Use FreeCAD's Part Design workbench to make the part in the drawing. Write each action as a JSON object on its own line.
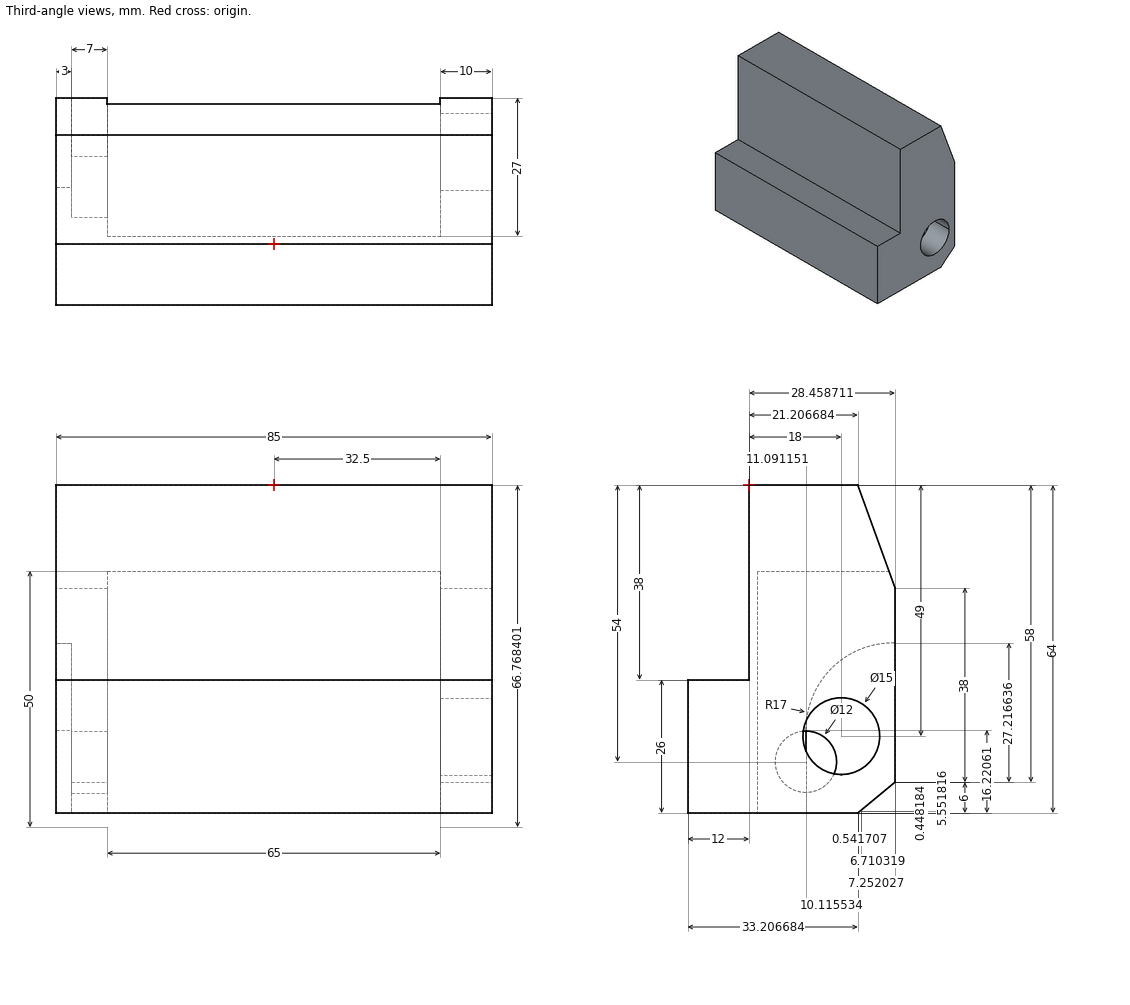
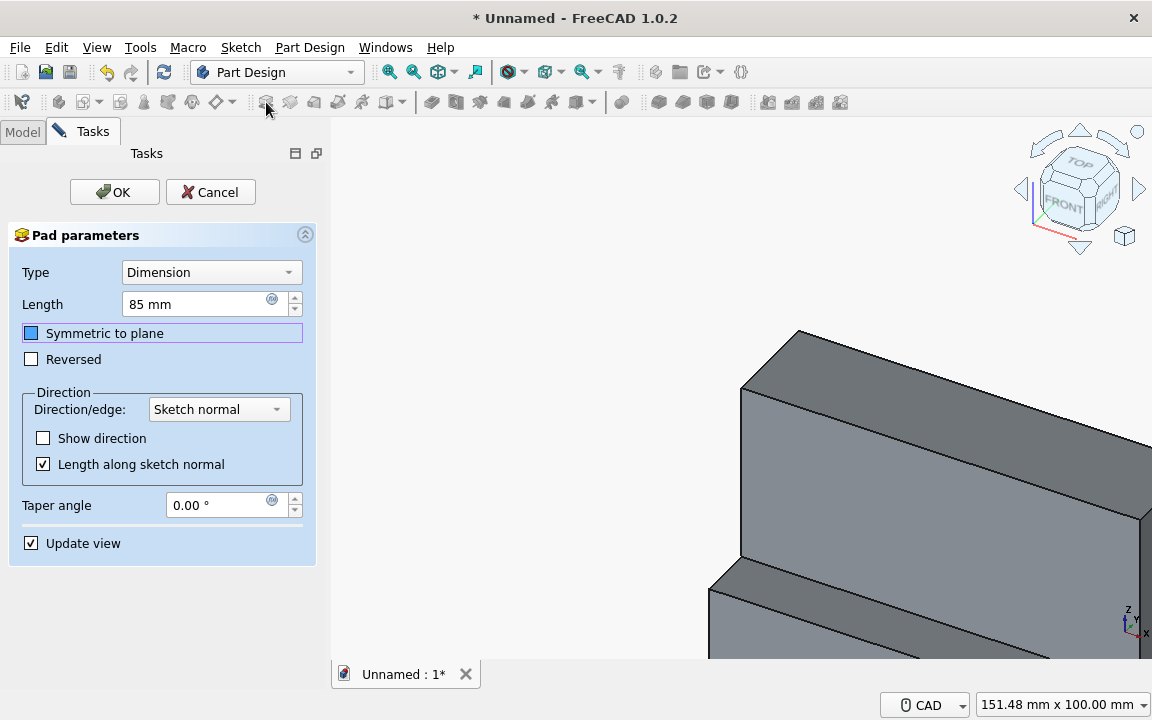
{"action": "left_click", "coordinate": [30, 333]}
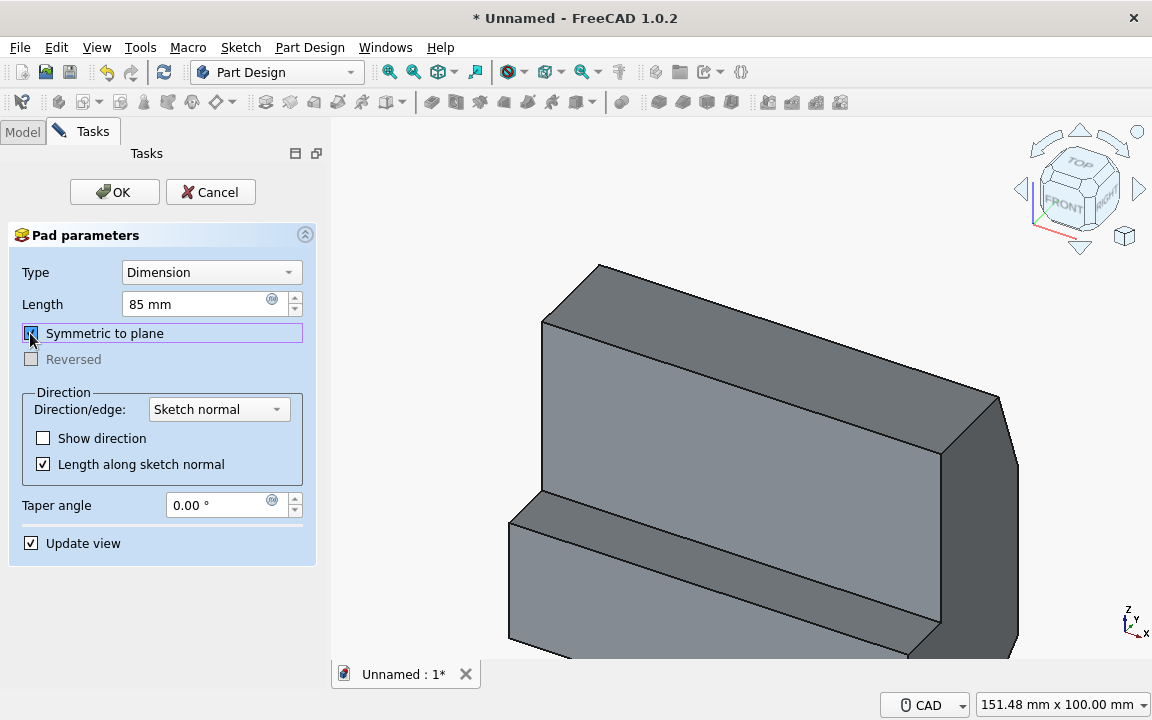
{"action": "left_click", "coordinate": [115, 192]}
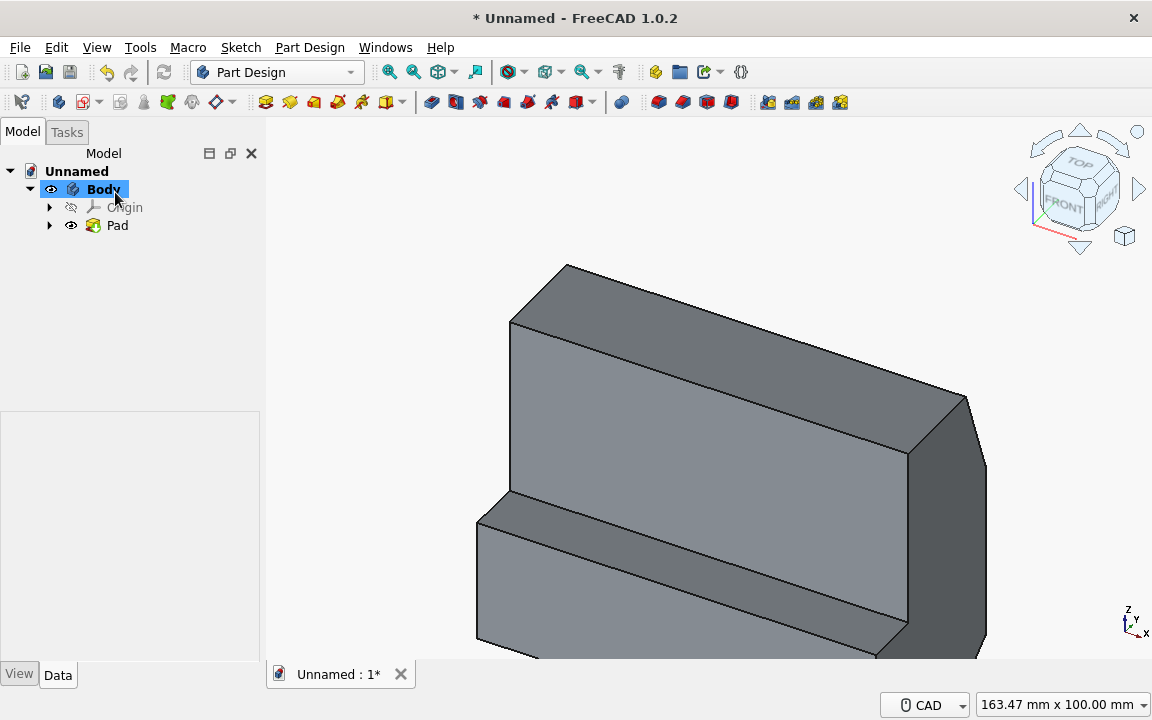
{"action": "left_click", "coordinate": [390, 72]}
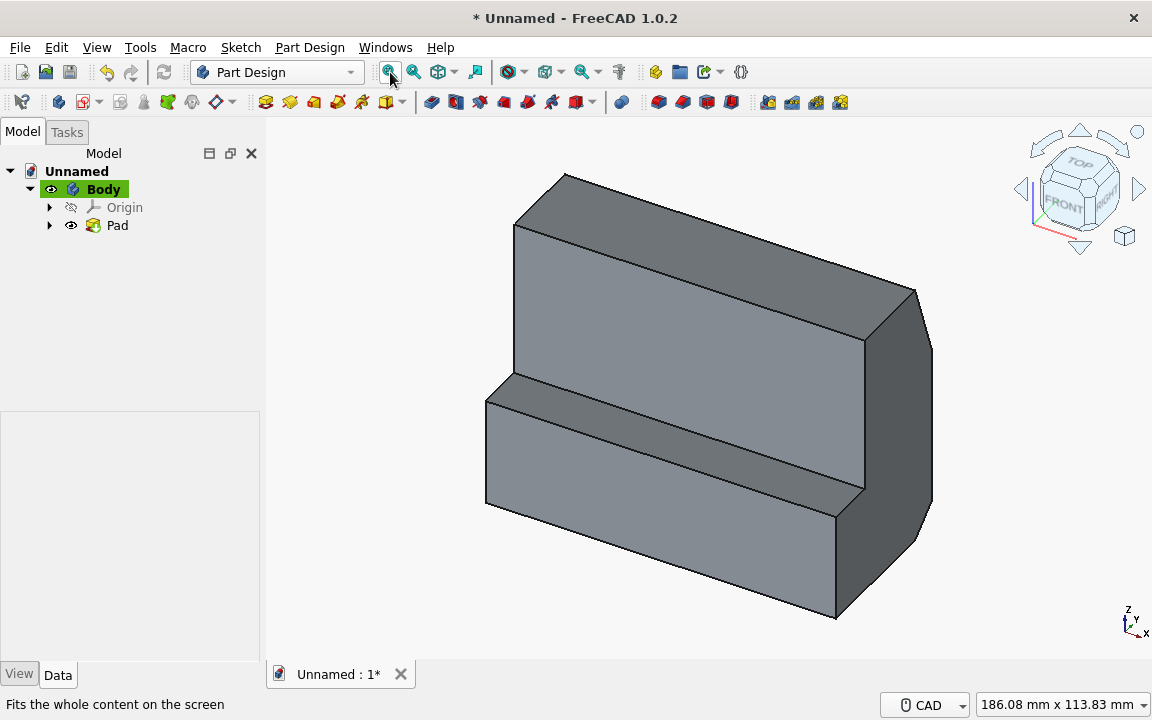
{"action": "key", "text": "4"}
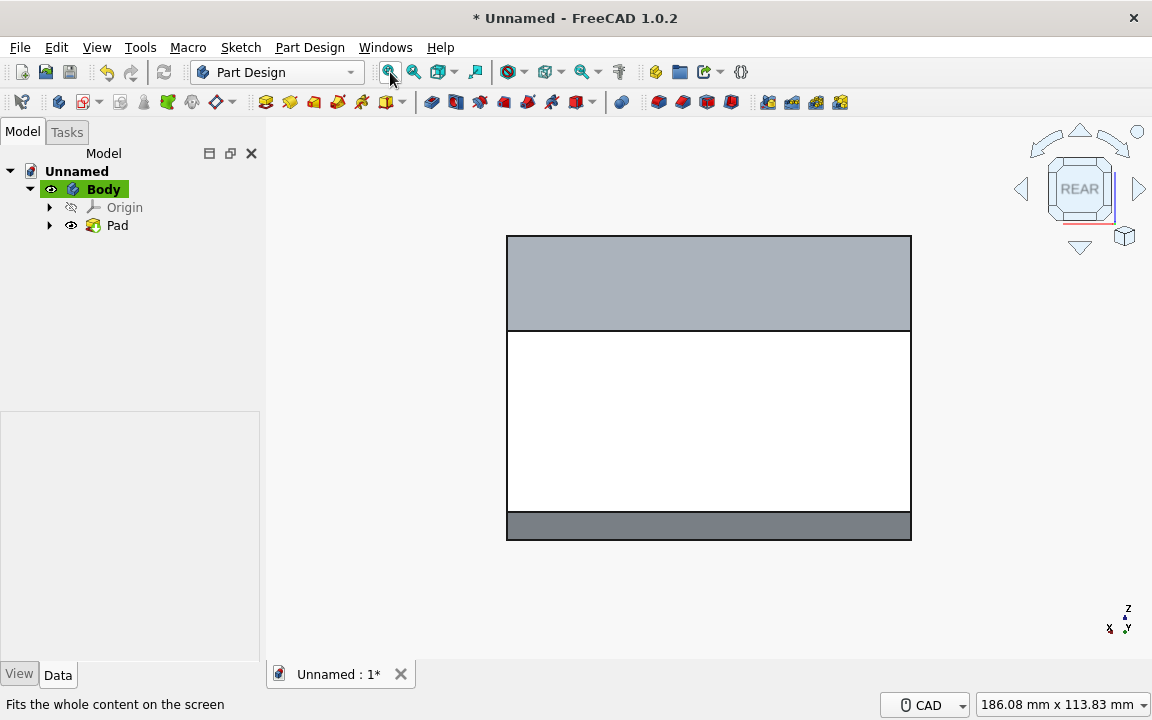
{"action": "left_click", "coordinate": [651, 420]}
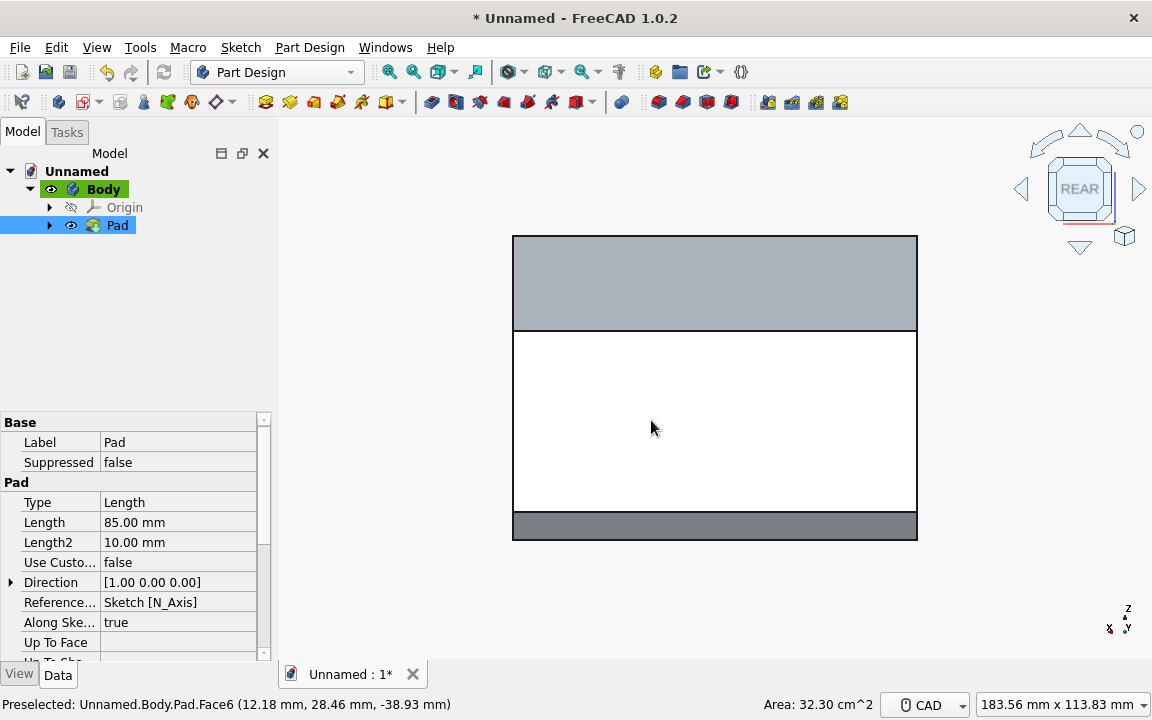
{"action": "left_click", "coordinate": [84, 102]}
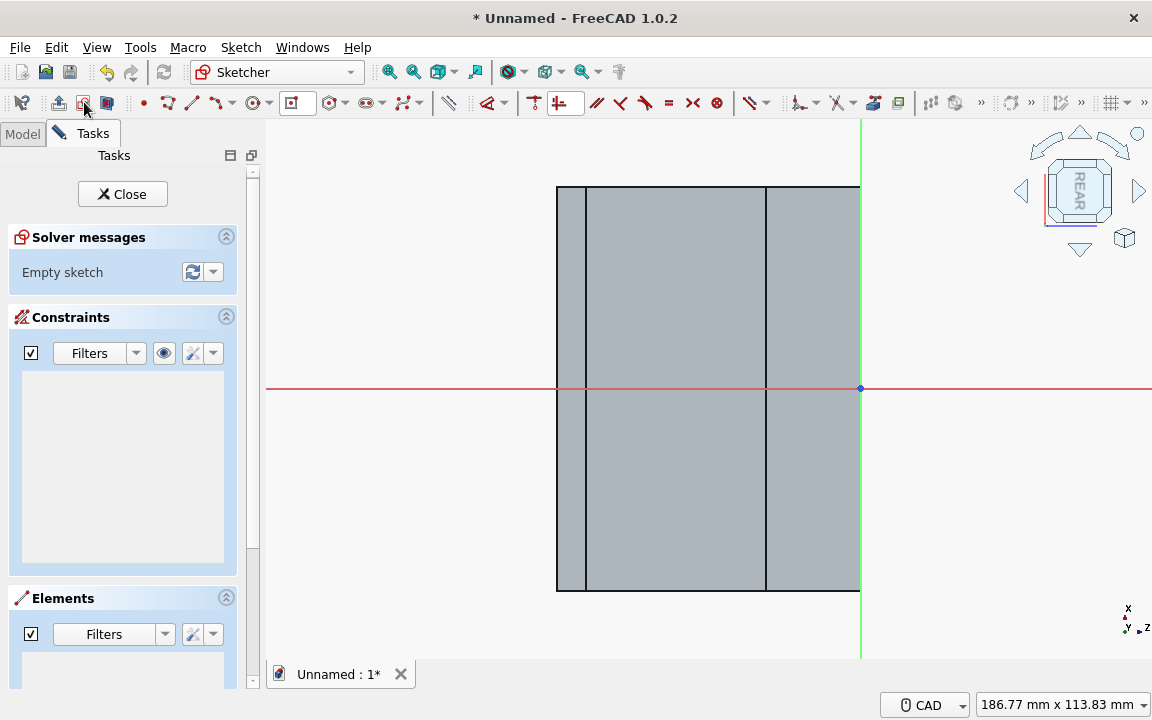
{"action": "key", "text": "g r"}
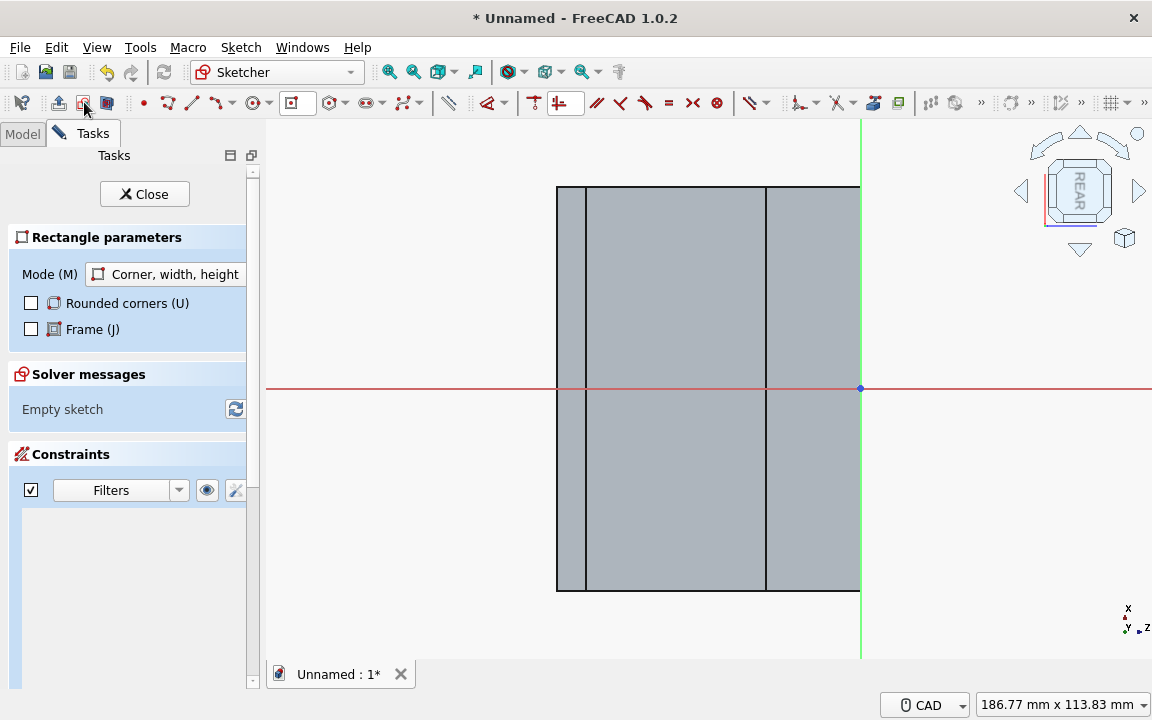
{"action": "left_click", "coordinate": [544, 235]}
{"action": "left_click", "coordinate": [781, 543]}
{"action": "key", "text": "Escape"}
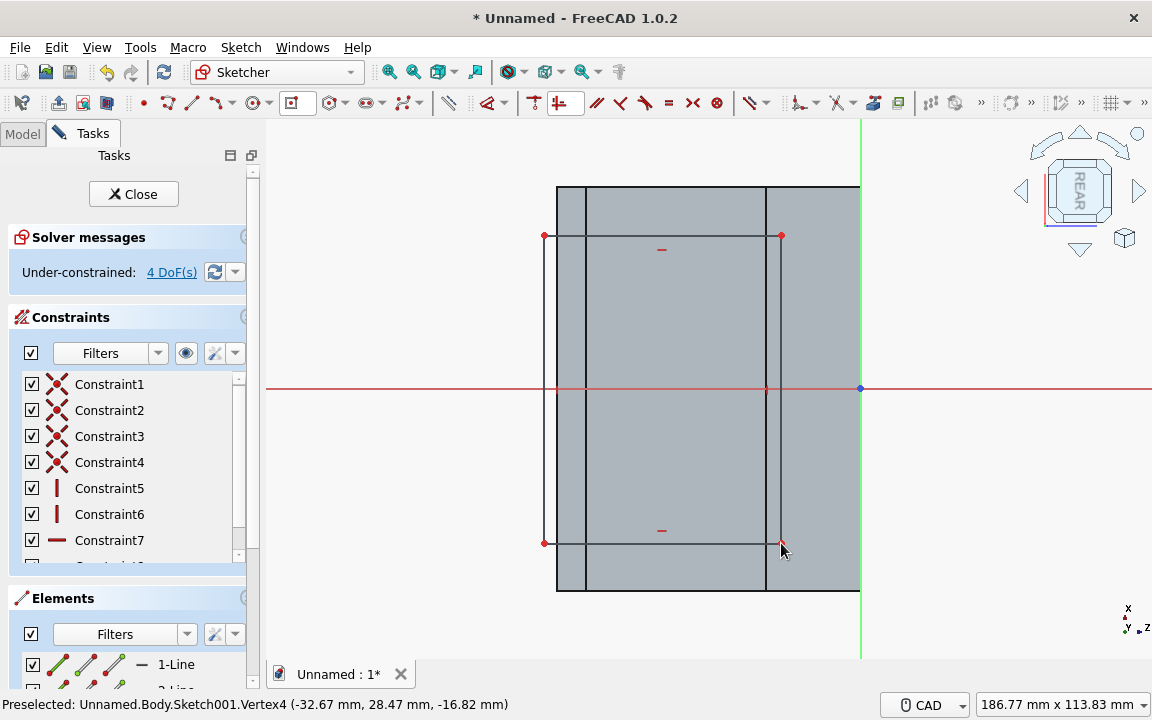
{"action": "left_click", "coordinate": [488, 104]}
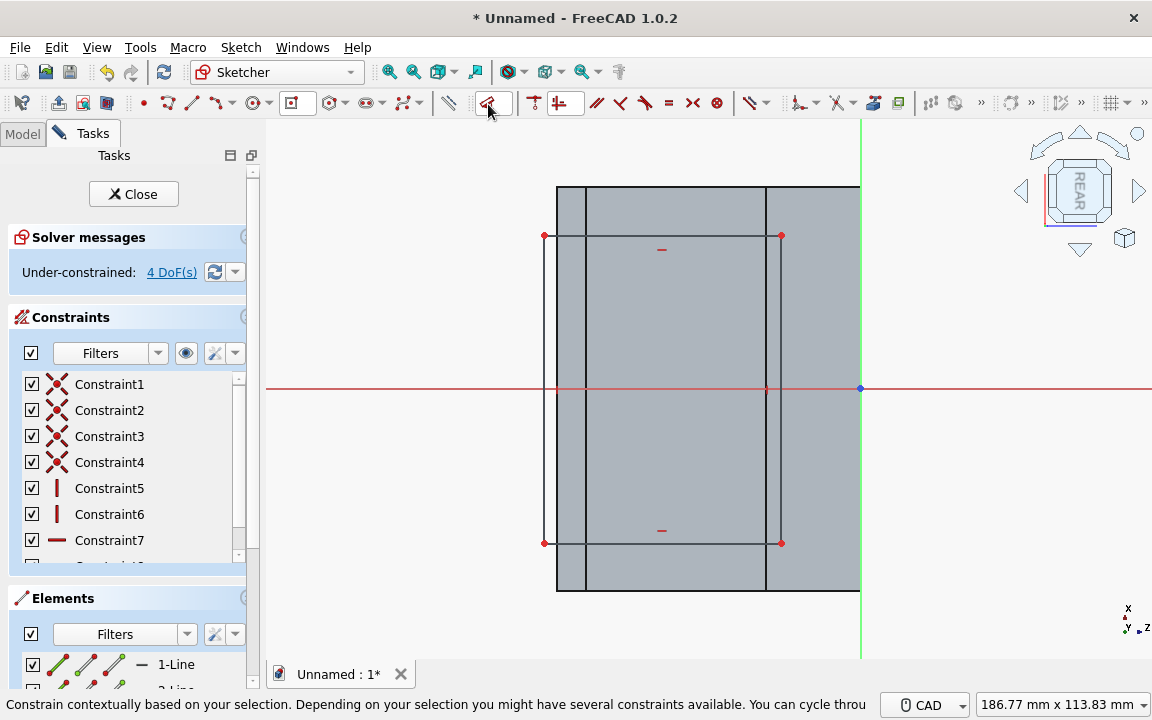
{"action": "left_click", "coordinate": [544, 328]}
{"action": "left_click", "coordinate": [510, 319]}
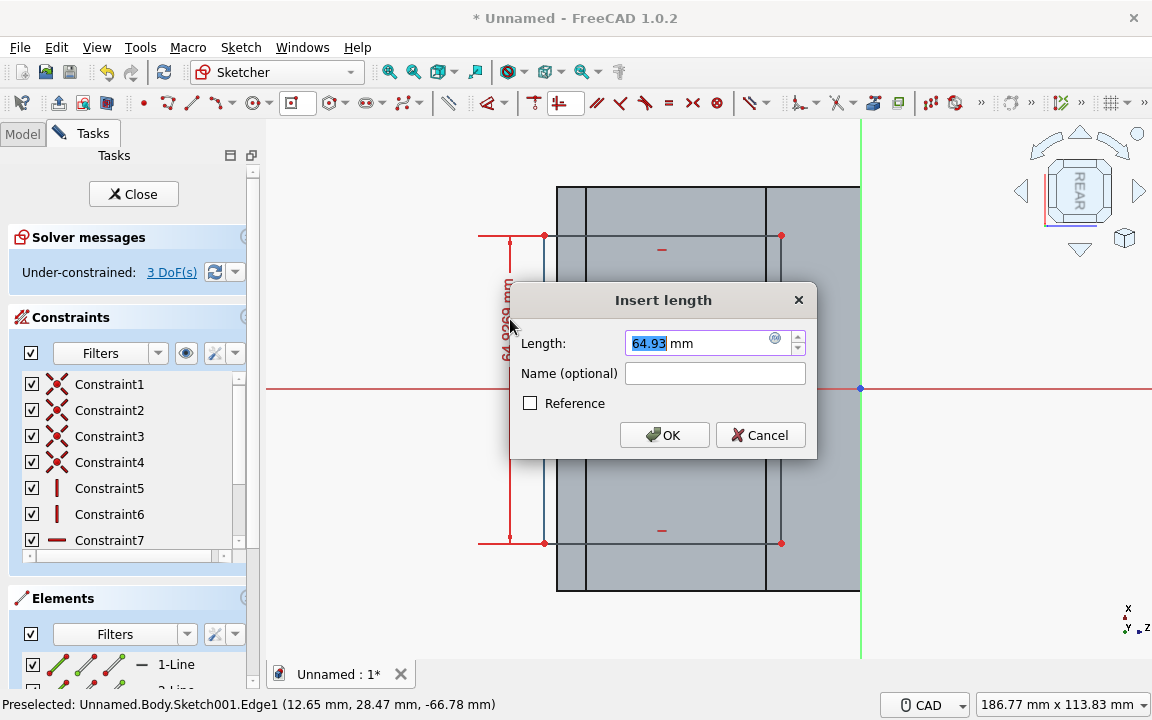
{"action": "type", "text": "65"}
{"action": "key", "text": "Return"}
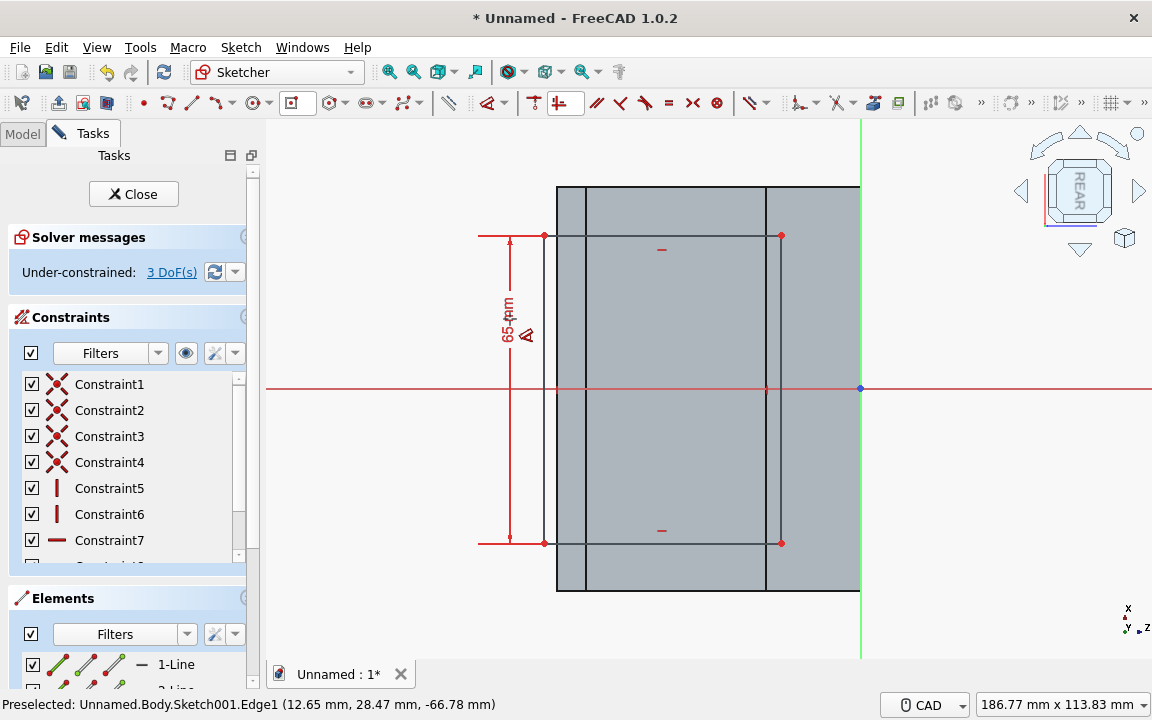
{"action": "left_click", "coordinate": [615, 544]}
{"action": "left_click", "coordinate": [662, 578]}